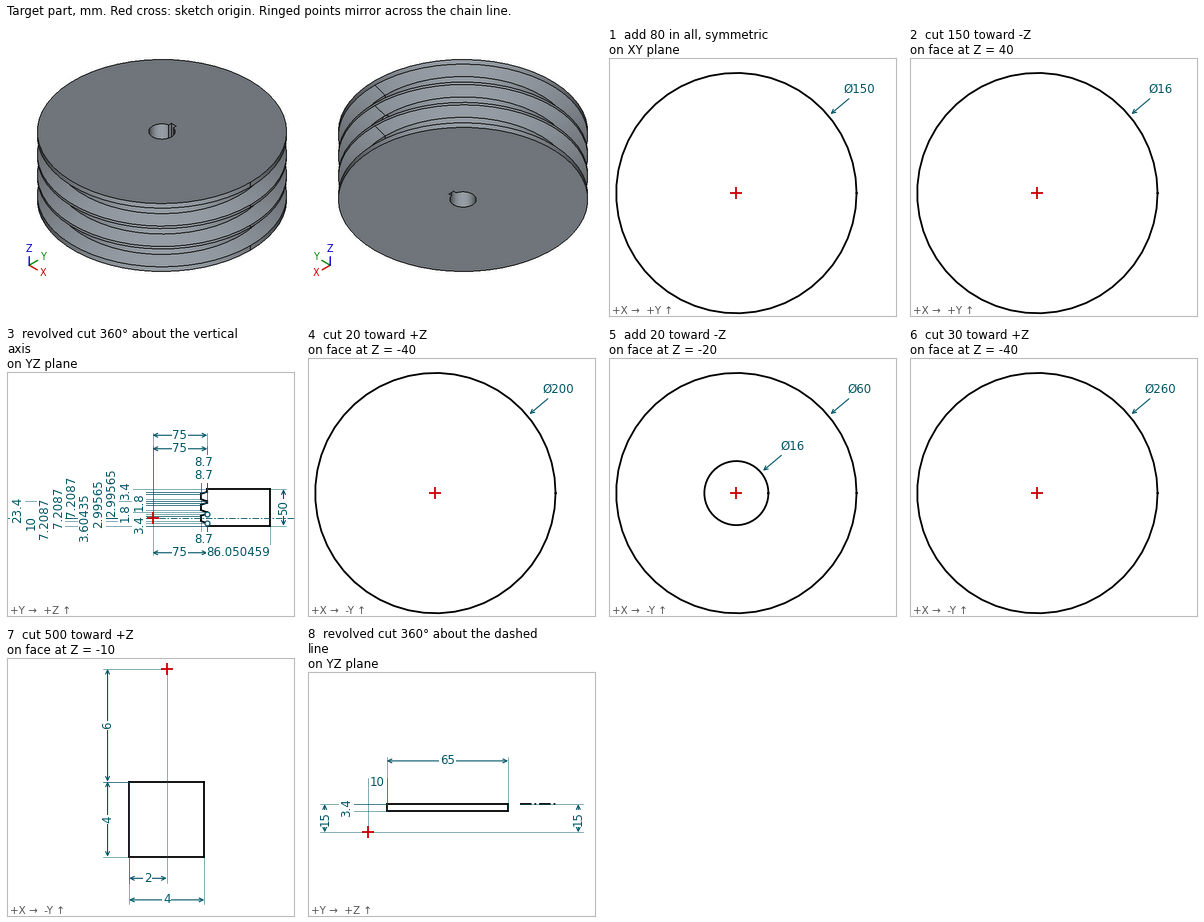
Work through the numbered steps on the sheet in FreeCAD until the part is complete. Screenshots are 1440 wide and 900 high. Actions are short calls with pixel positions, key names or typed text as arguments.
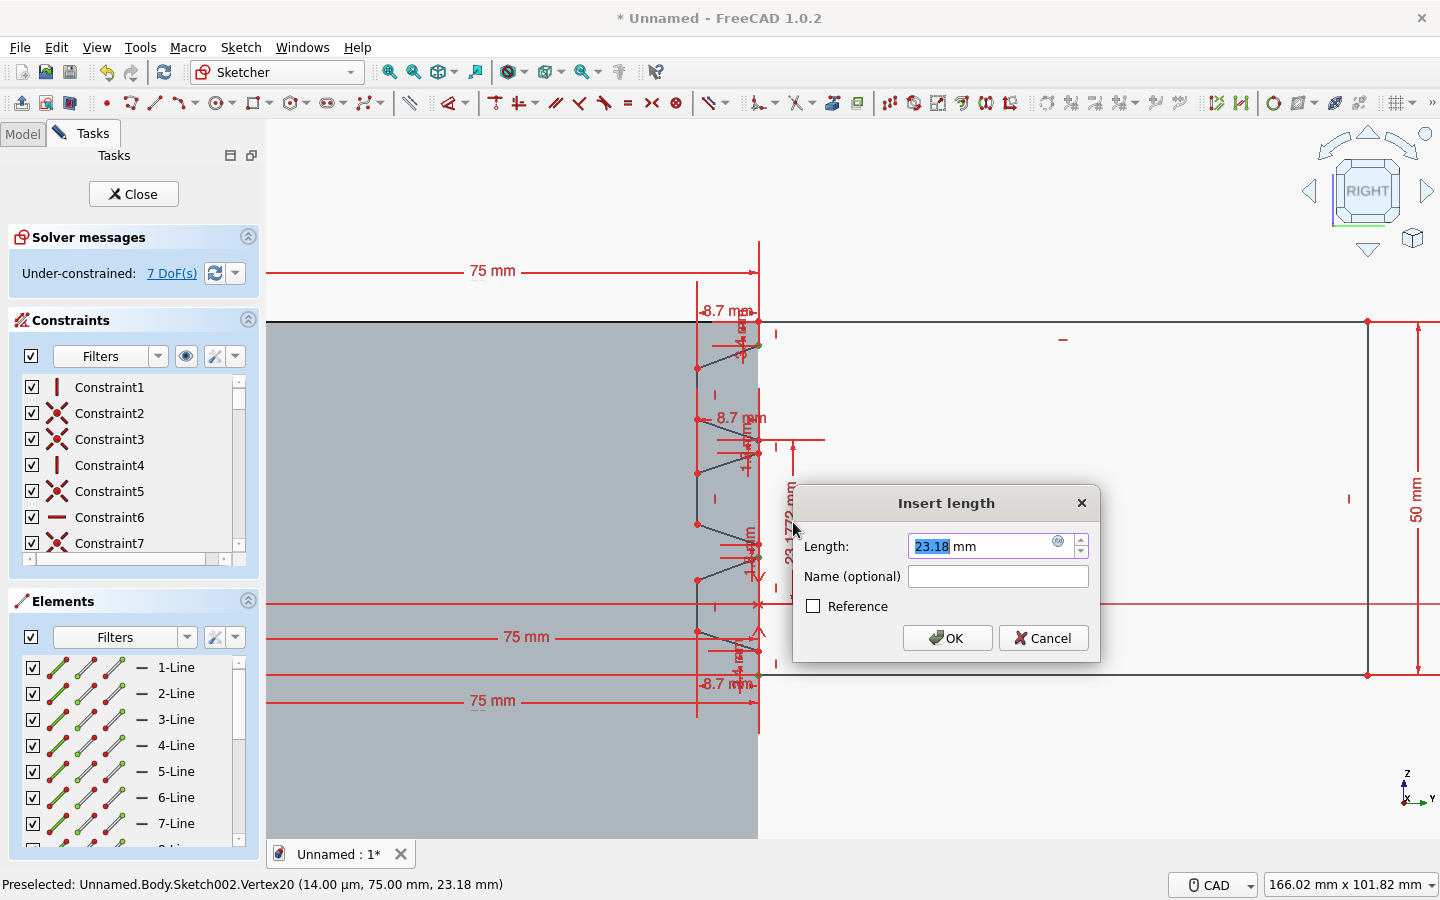
text(23.4)
key(Return)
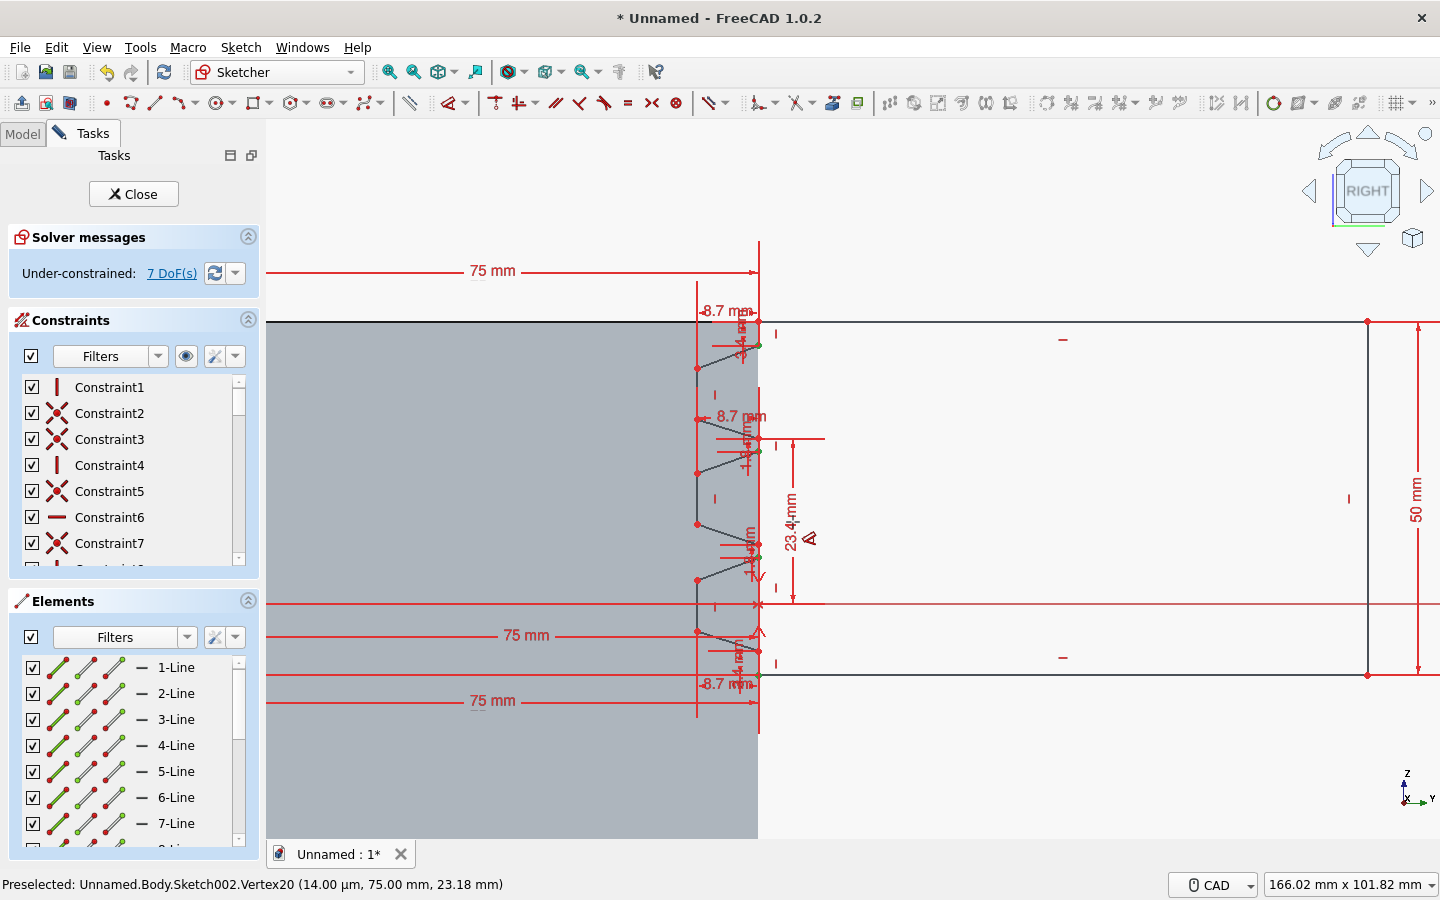
click(697, 616)
click(663, 618)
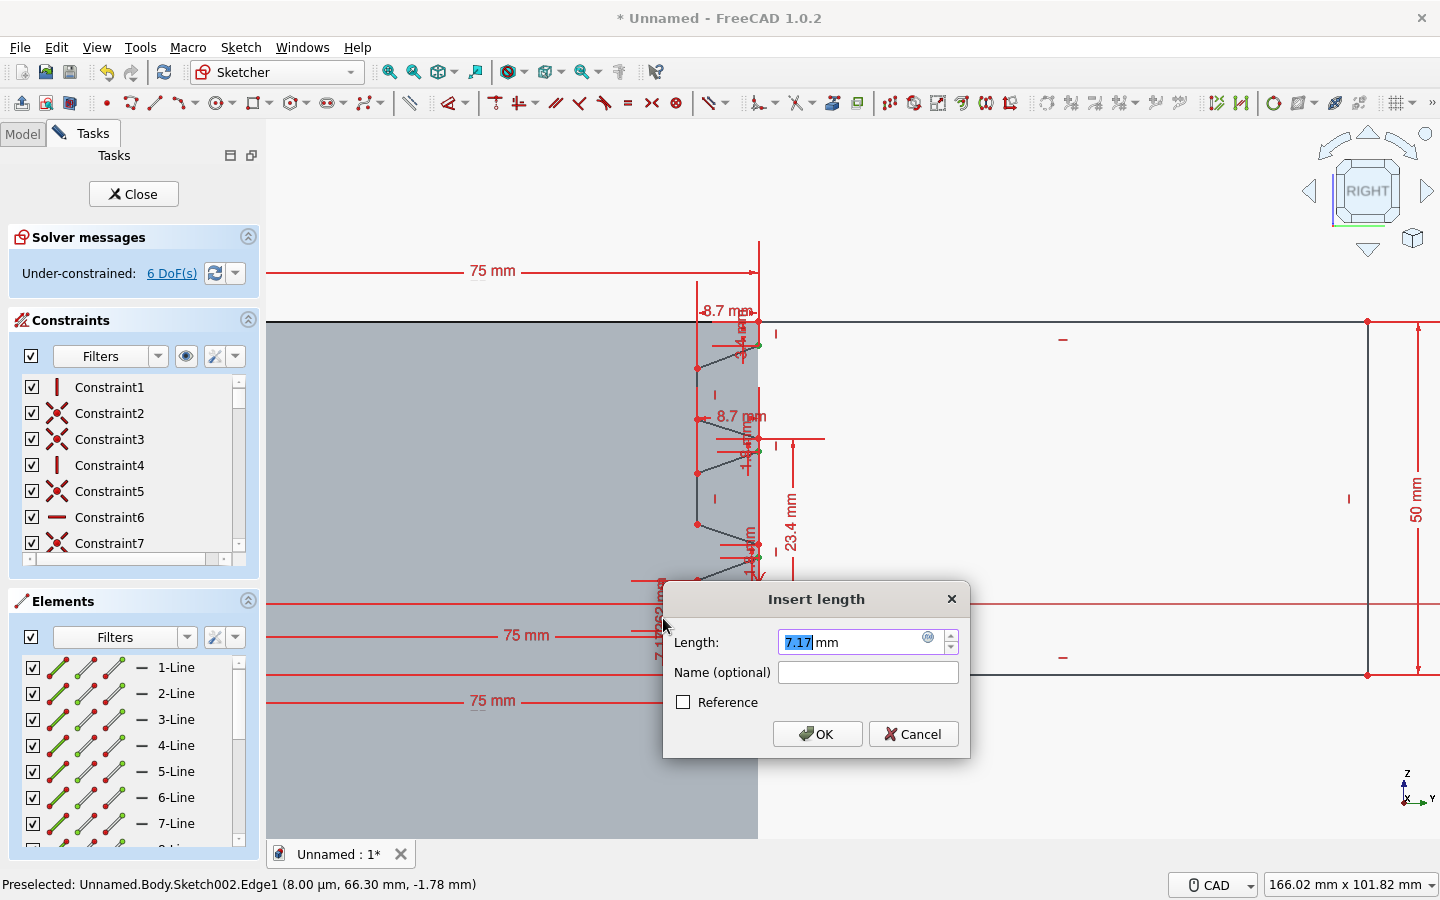
text(7.2087)
key(Return)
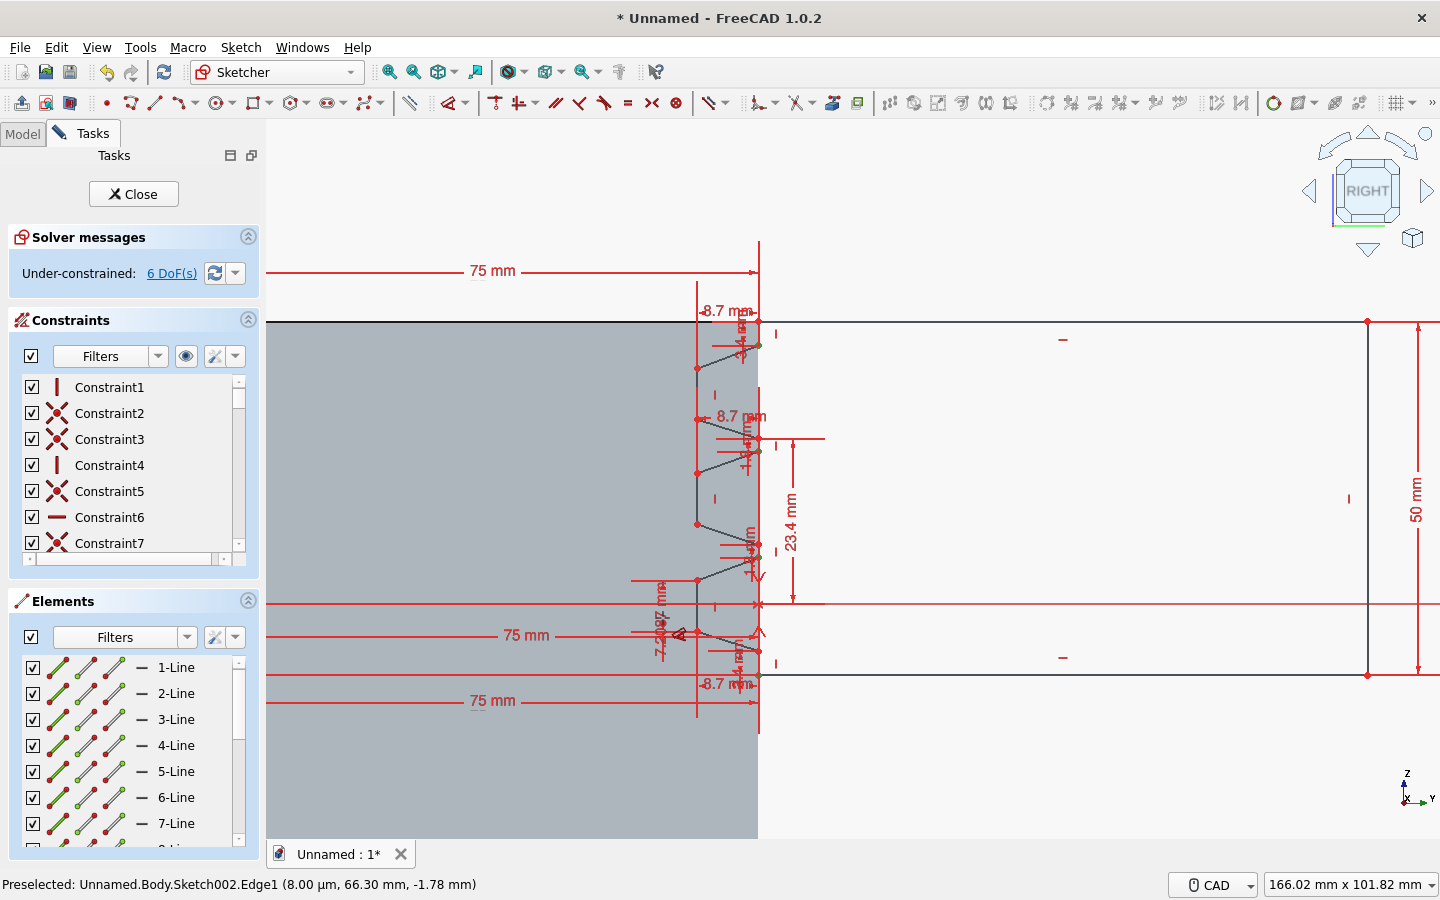
click(697, 384)
click(663, 394)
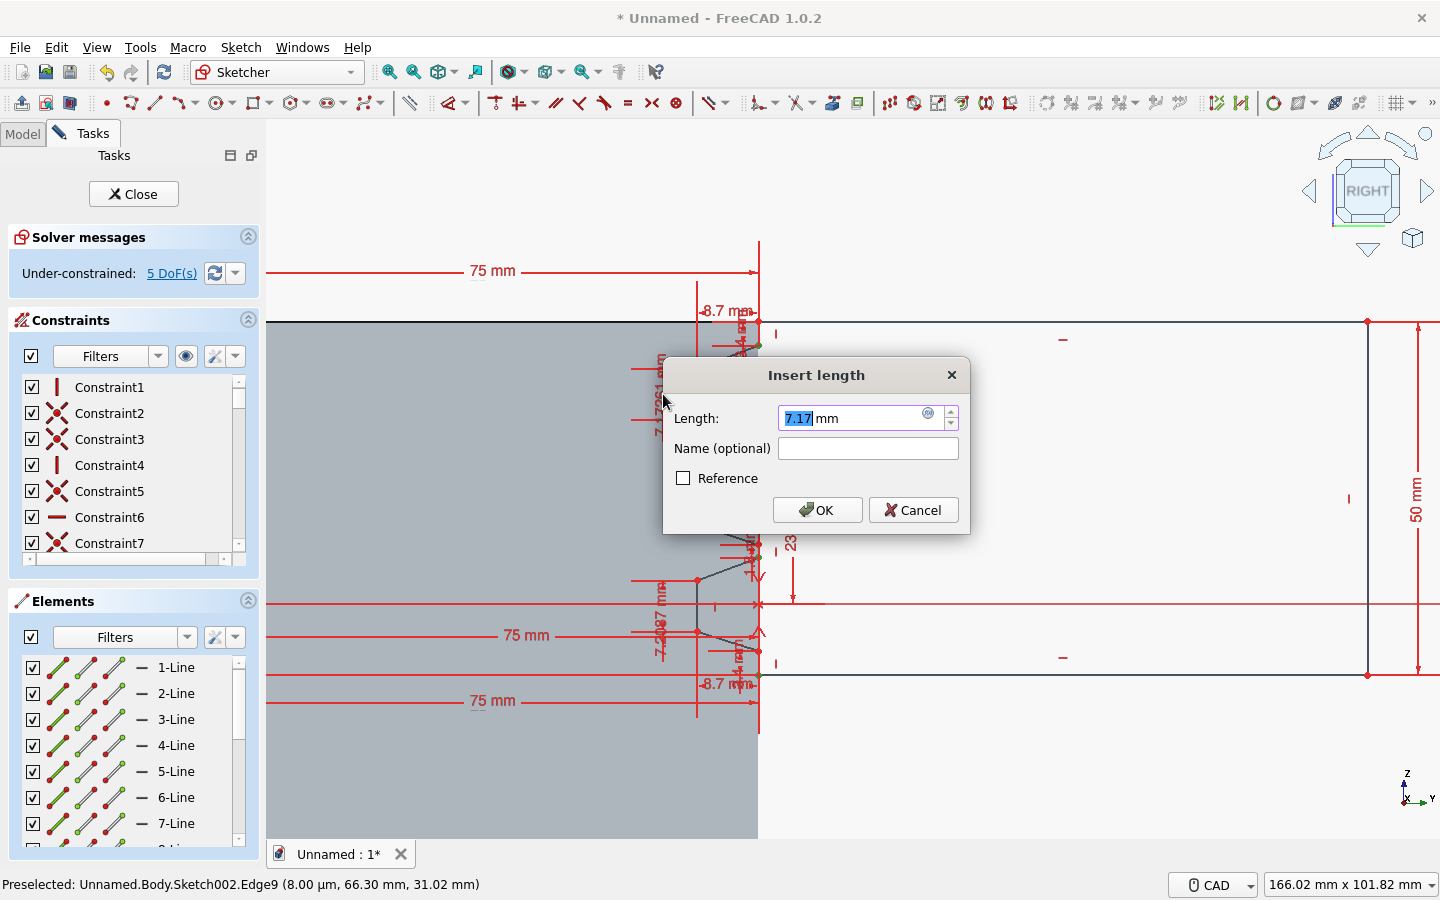
text(7.2087)
key(Return)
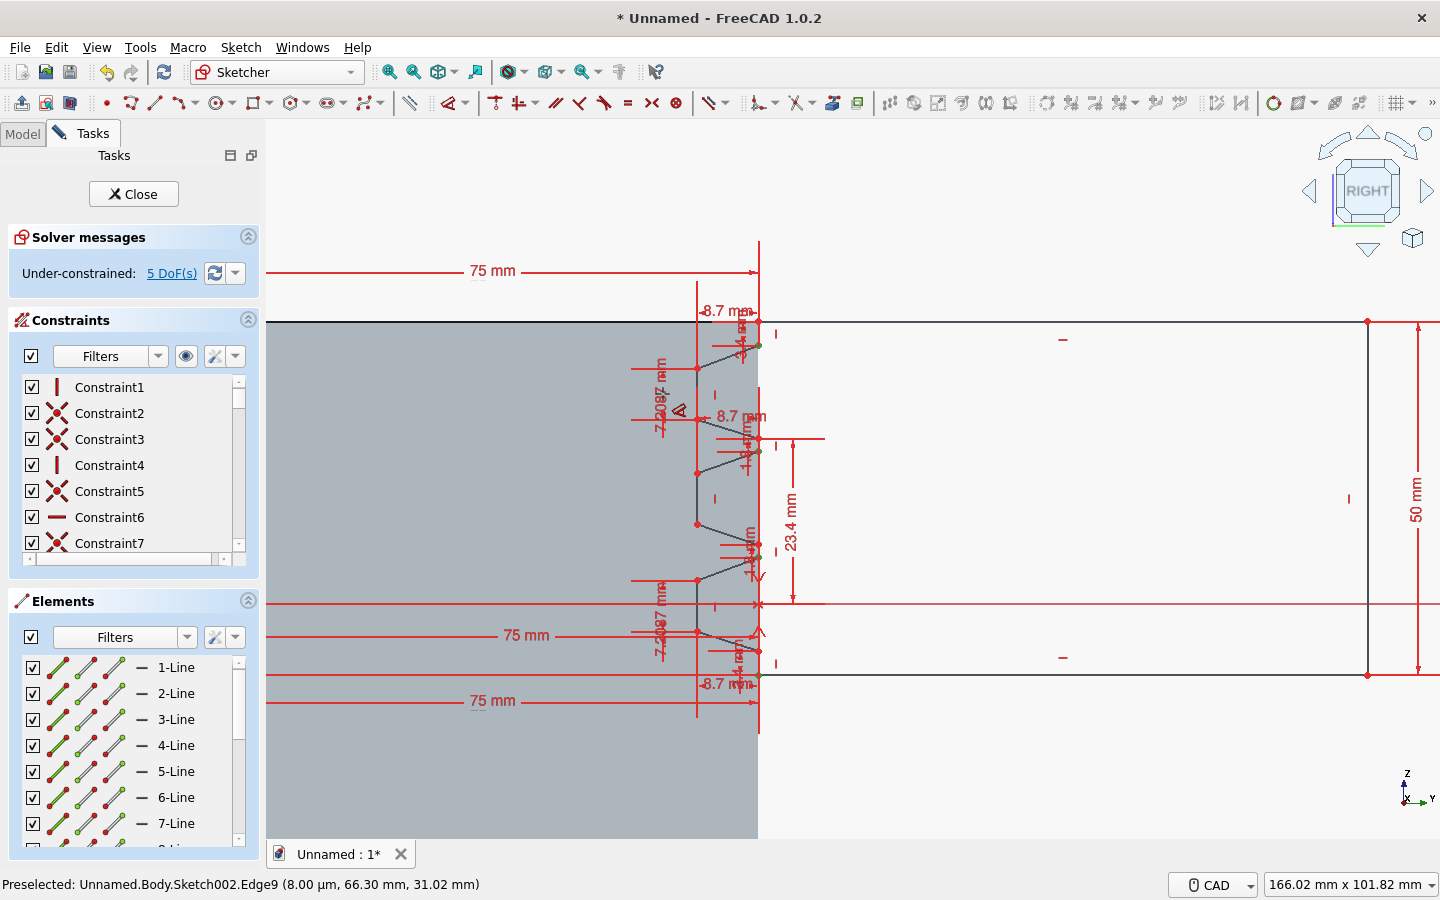
click(697, 489)
click(663, 499)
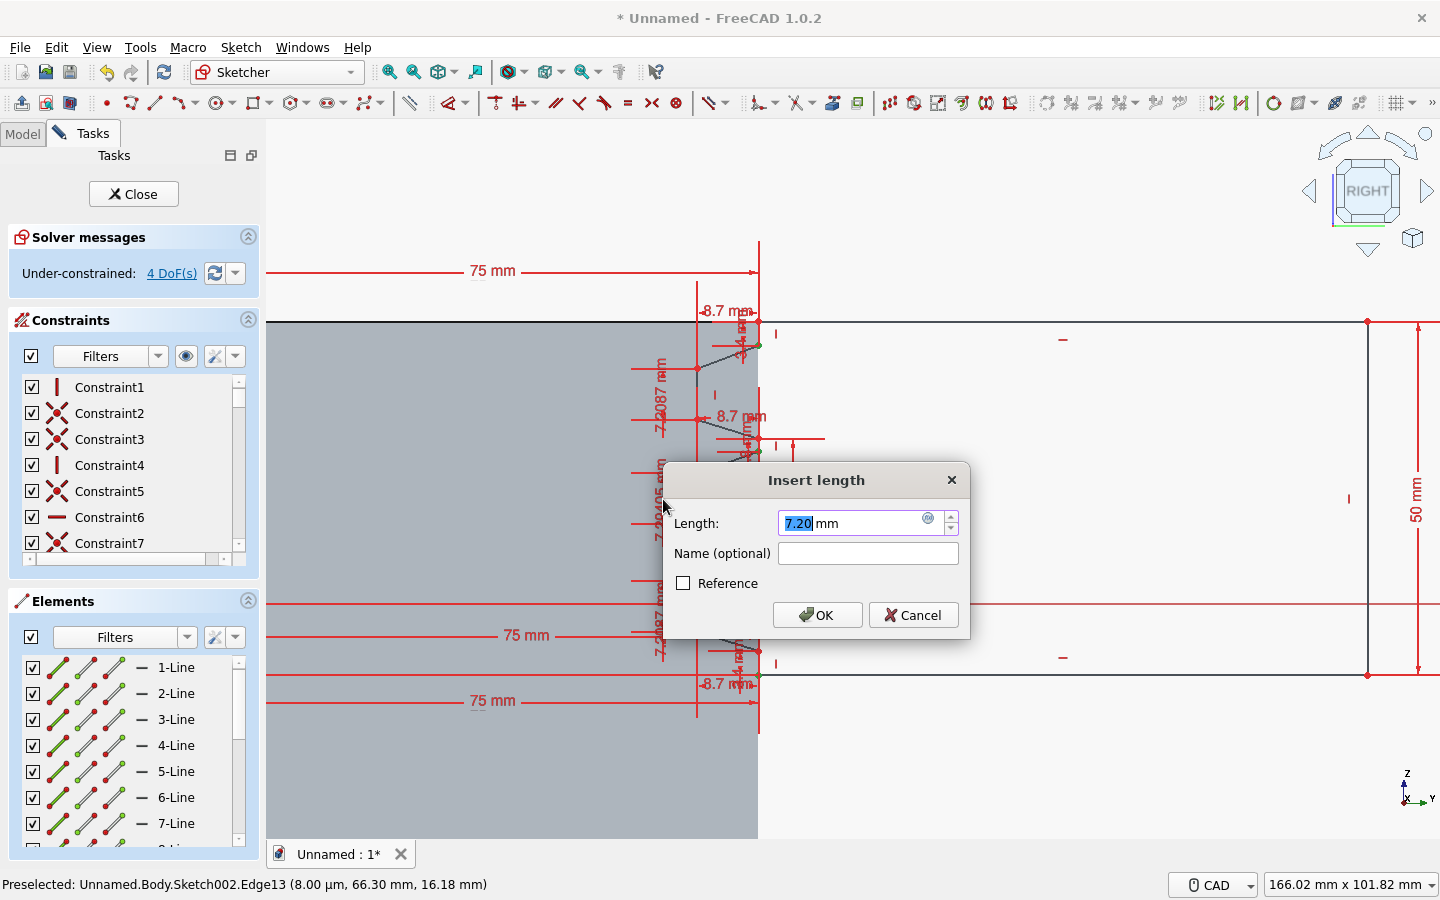
text(7.2087)
key(Return)